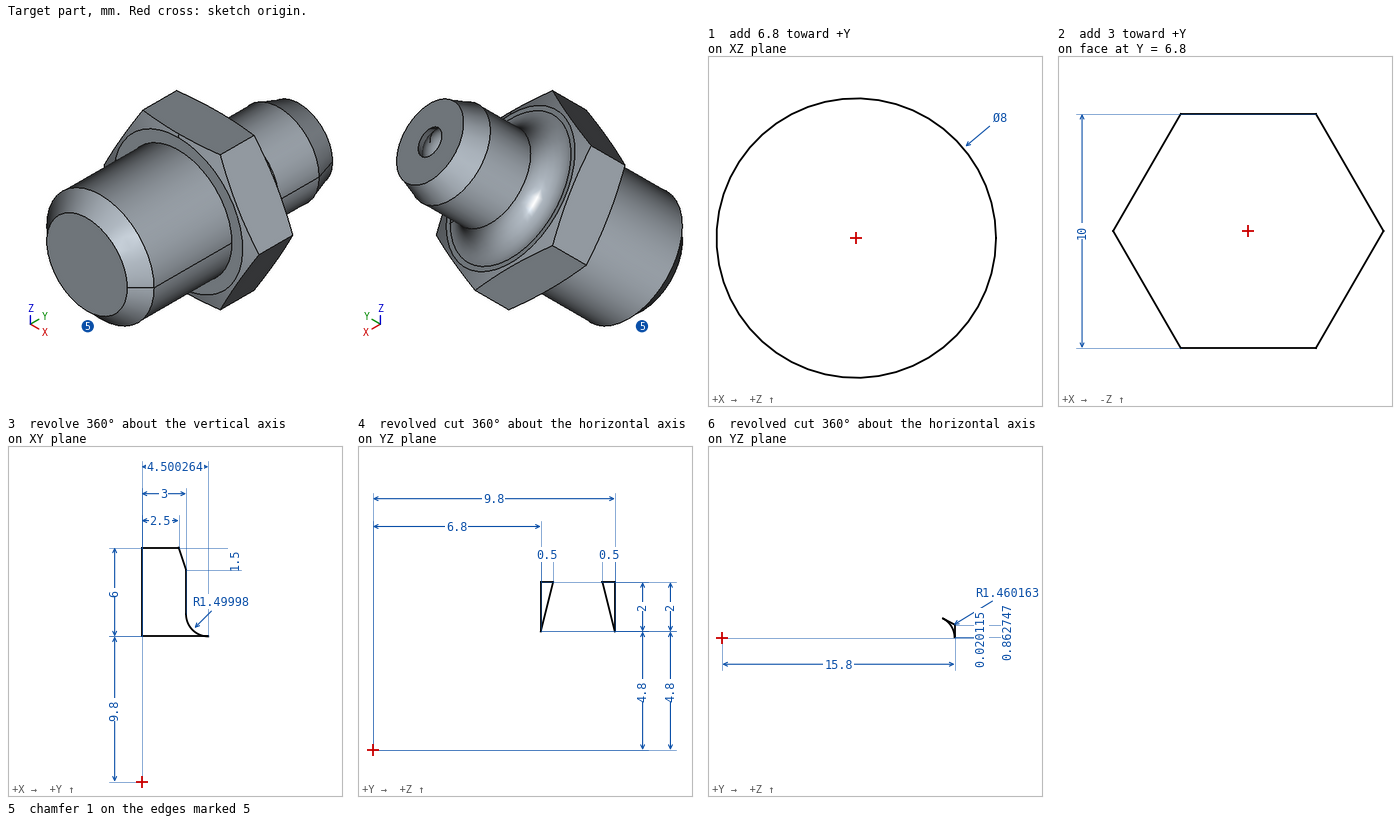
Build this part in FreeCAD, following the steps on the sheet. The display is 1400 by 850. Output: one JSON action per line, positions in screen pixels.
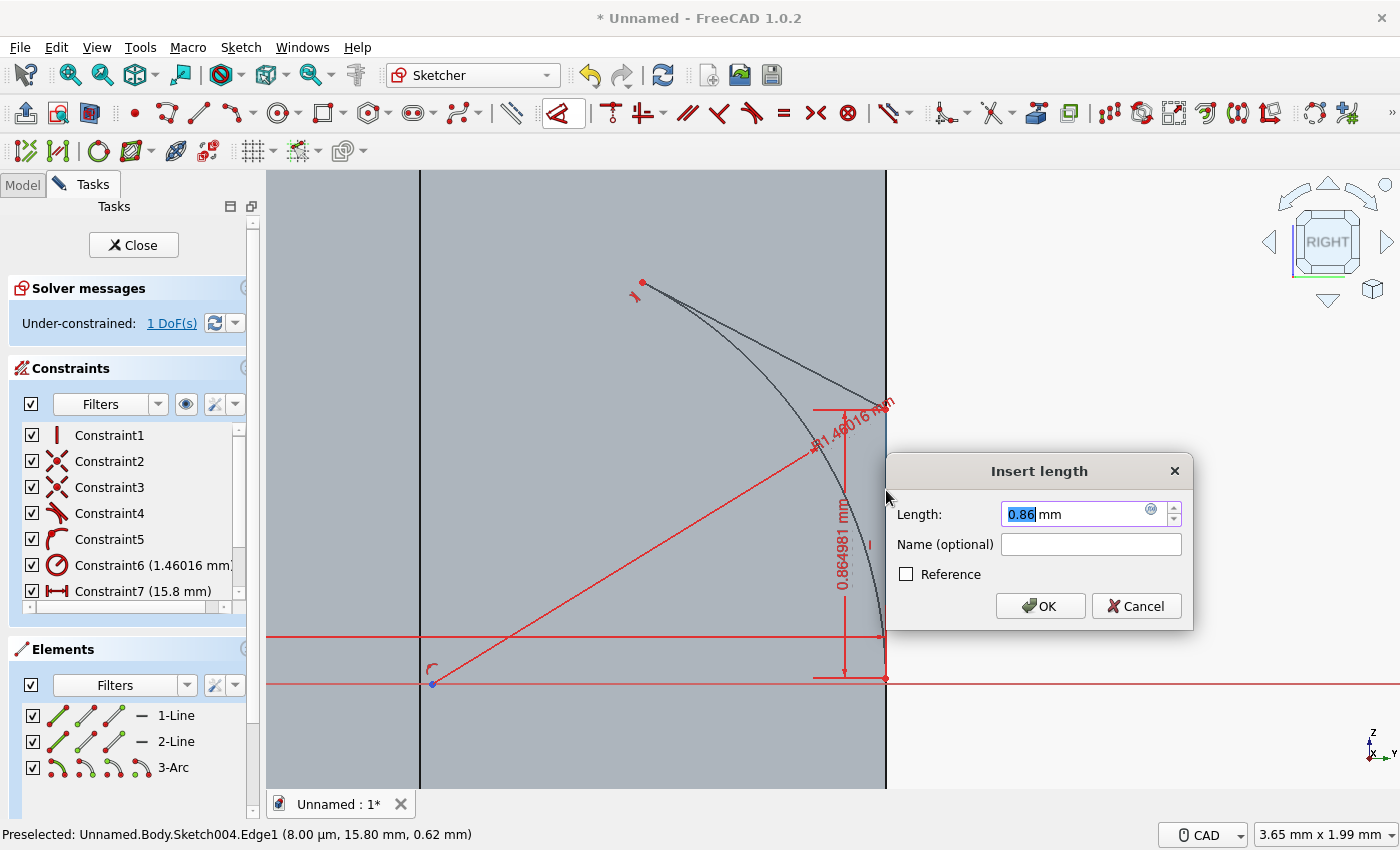
{"action": "type", "text": "0.862747"}
{"action": "key", "text": "Return"}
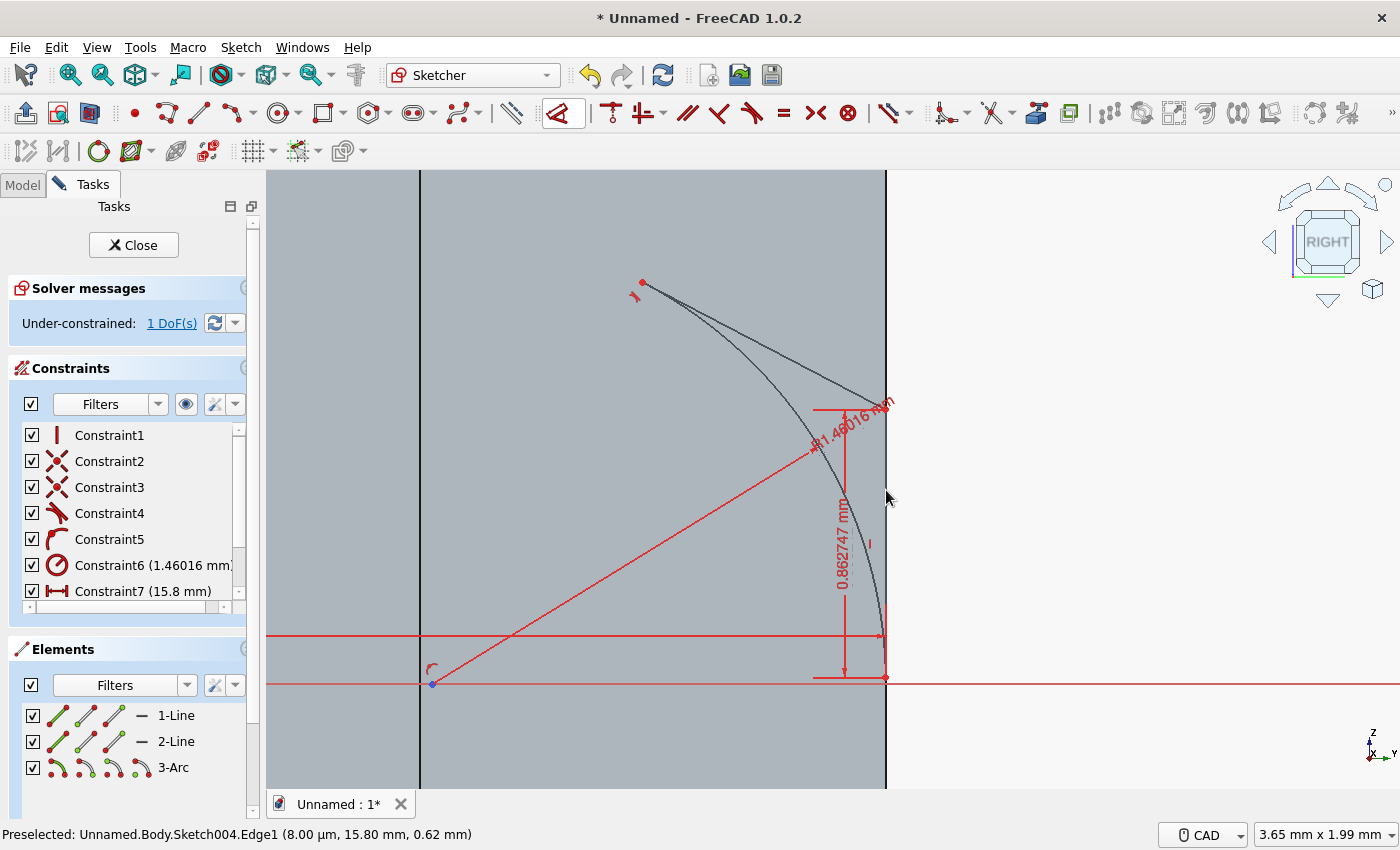
{"action": "scroll", "coordinate": [886, 678], "scroll_direction": "up", "scroll_amount": 10}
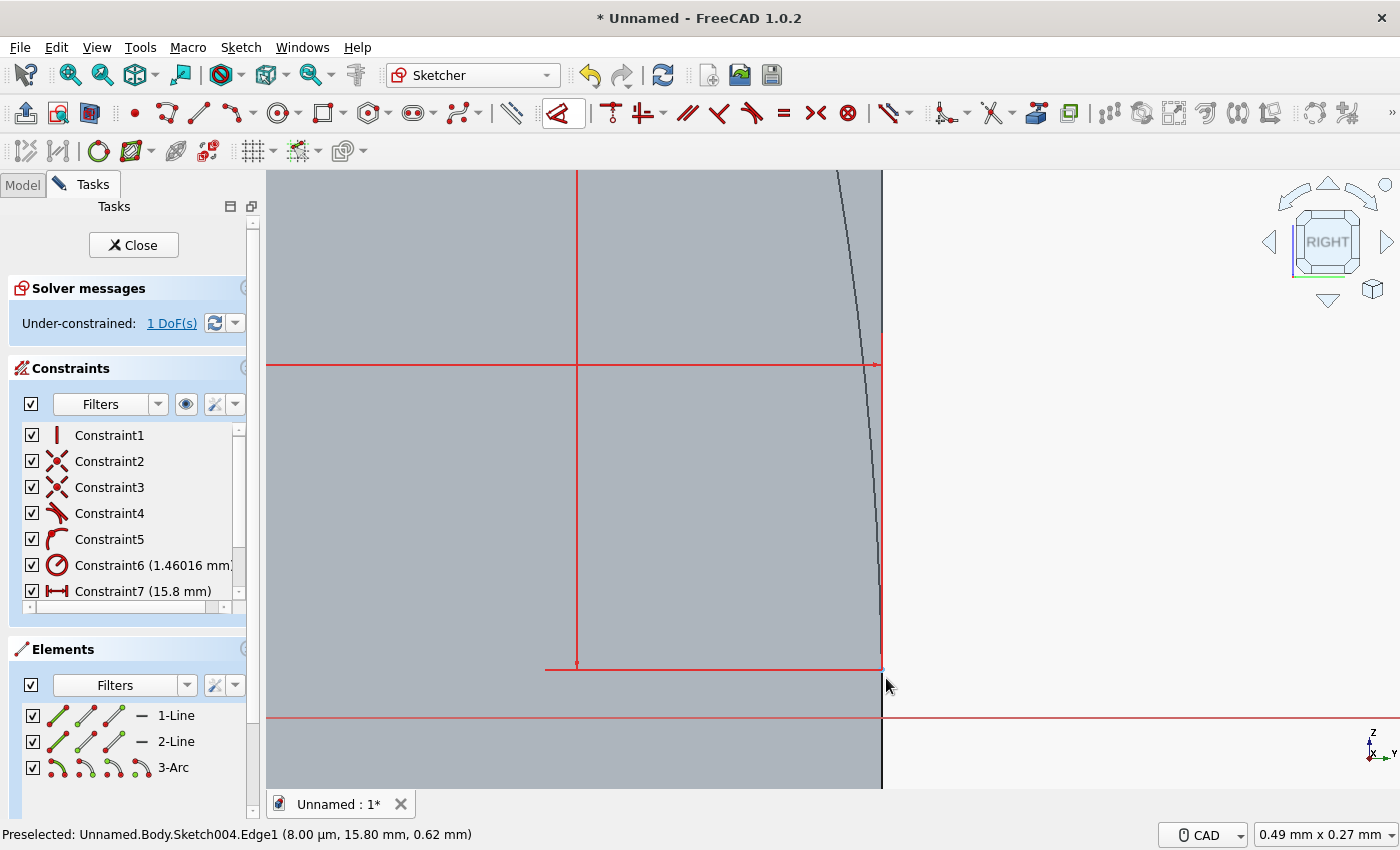
{"action": "left_click", "coordinate": [882, 670]}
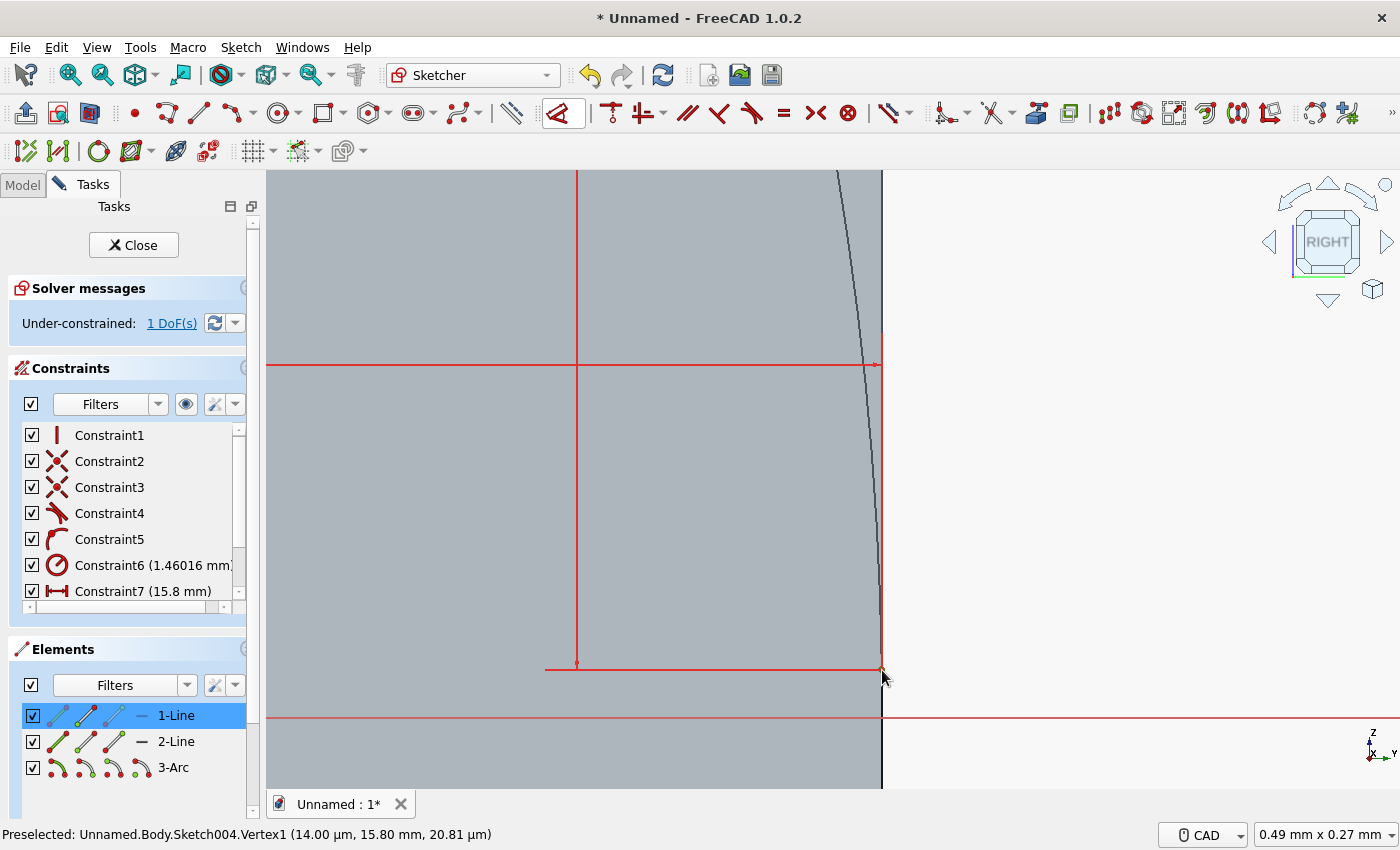
{"action": "key", "text": "i"}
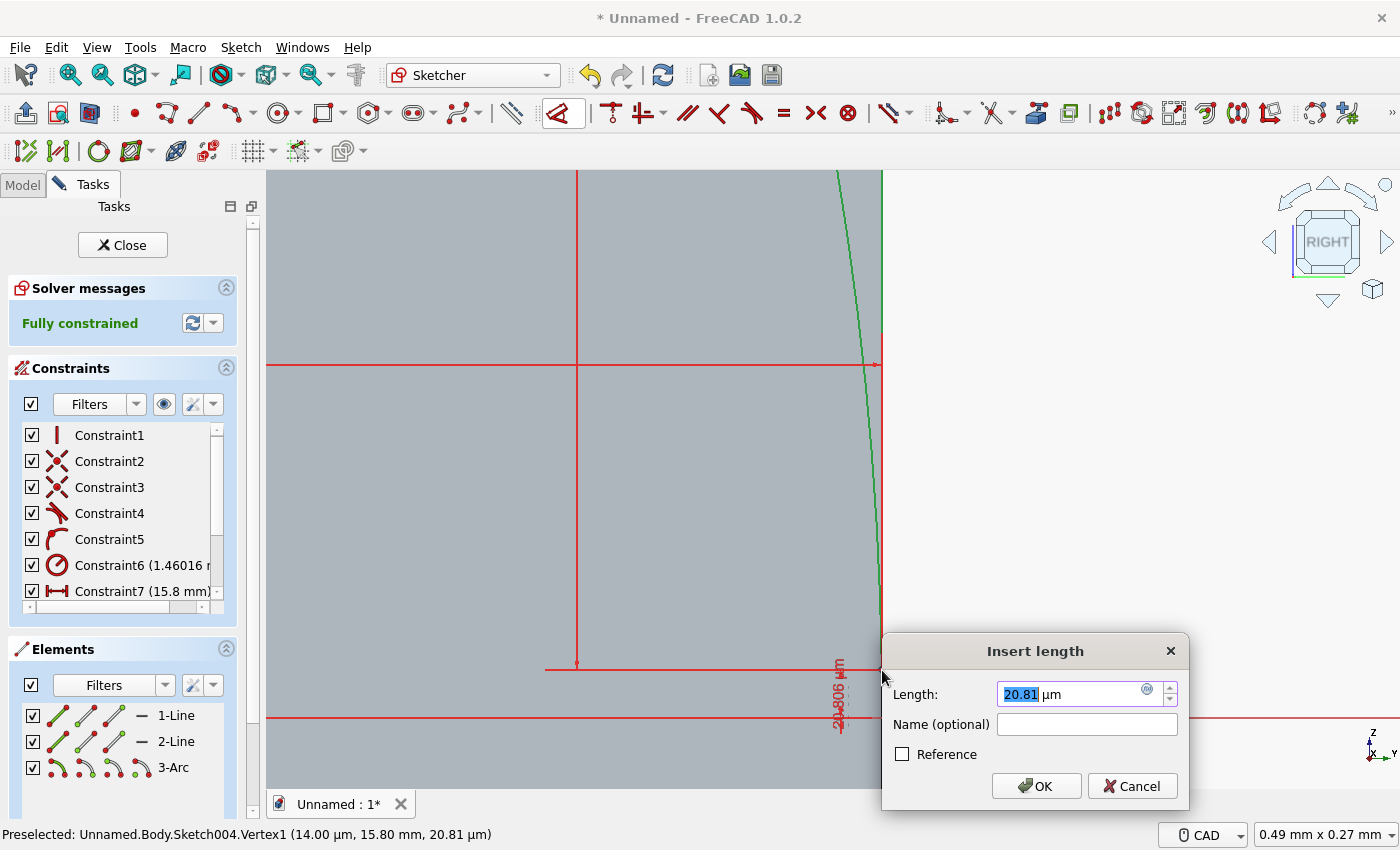
{"action": "key", "text": "ctrl+a"}
{"action": "type", "text": "0.020115 mm"}
{"action": "key", "text": "Return"}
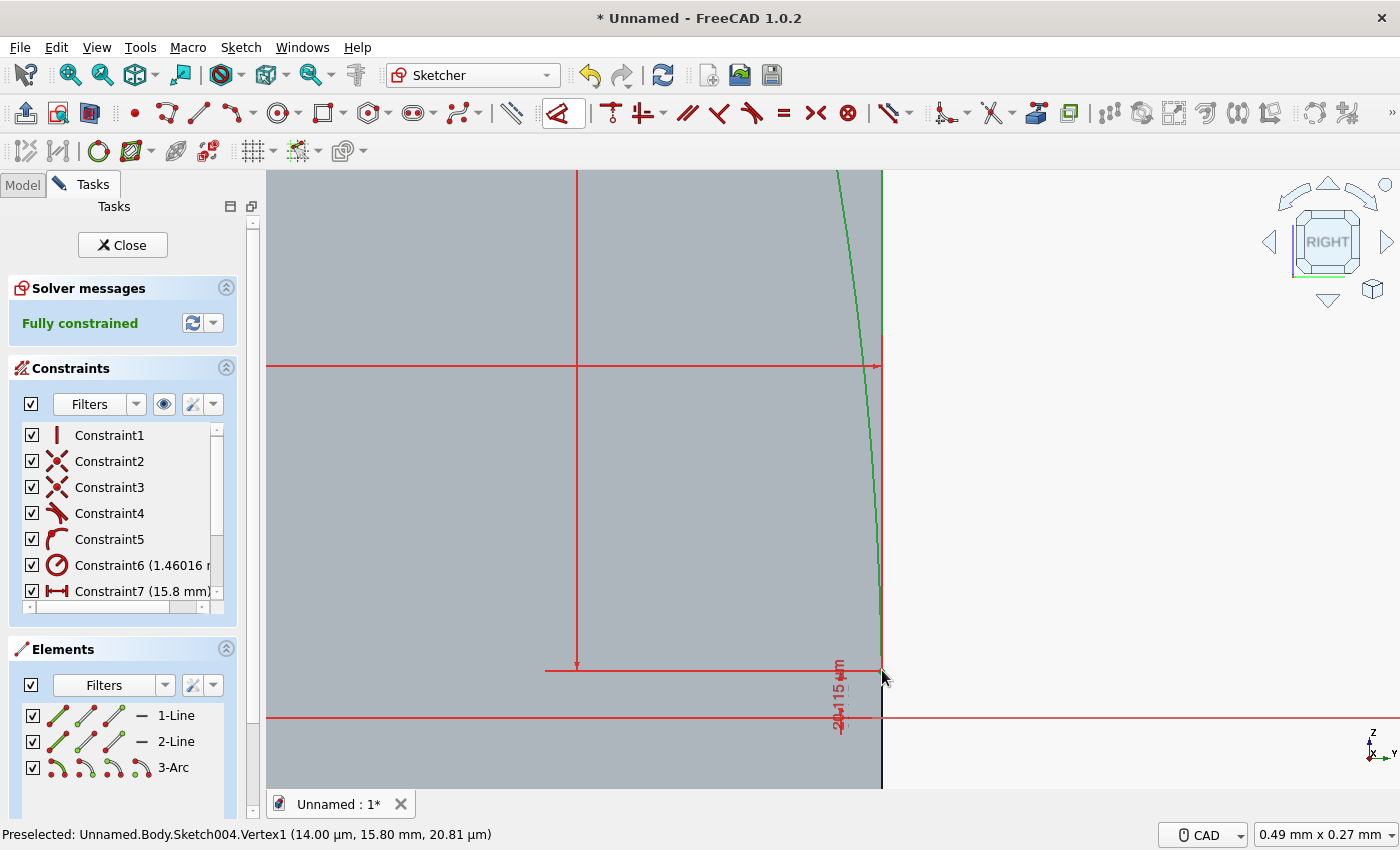
{"action": "left_click", "coordinate": [123, 245]}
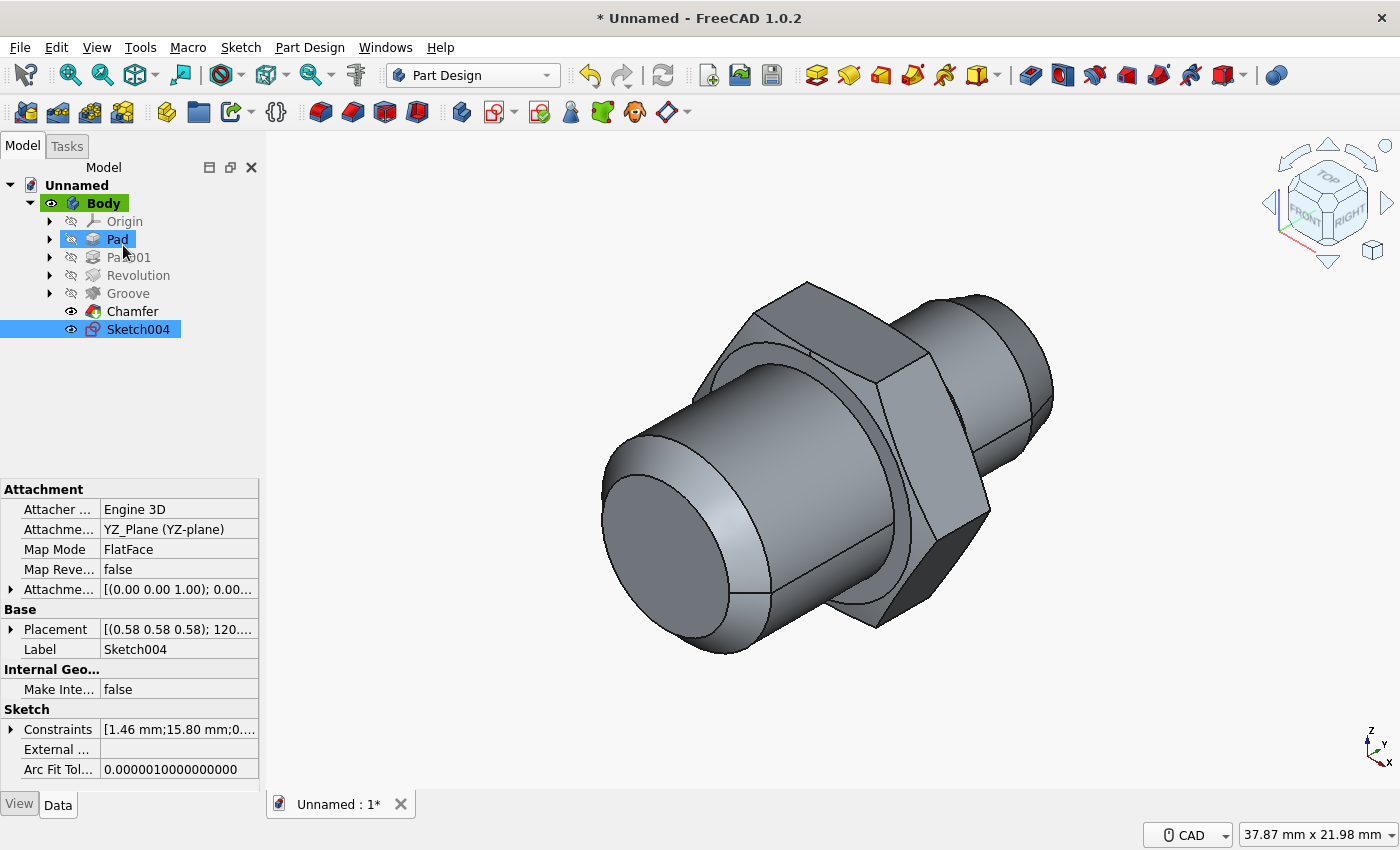
{"action": "left_click", "coordinate": [1096, 76]}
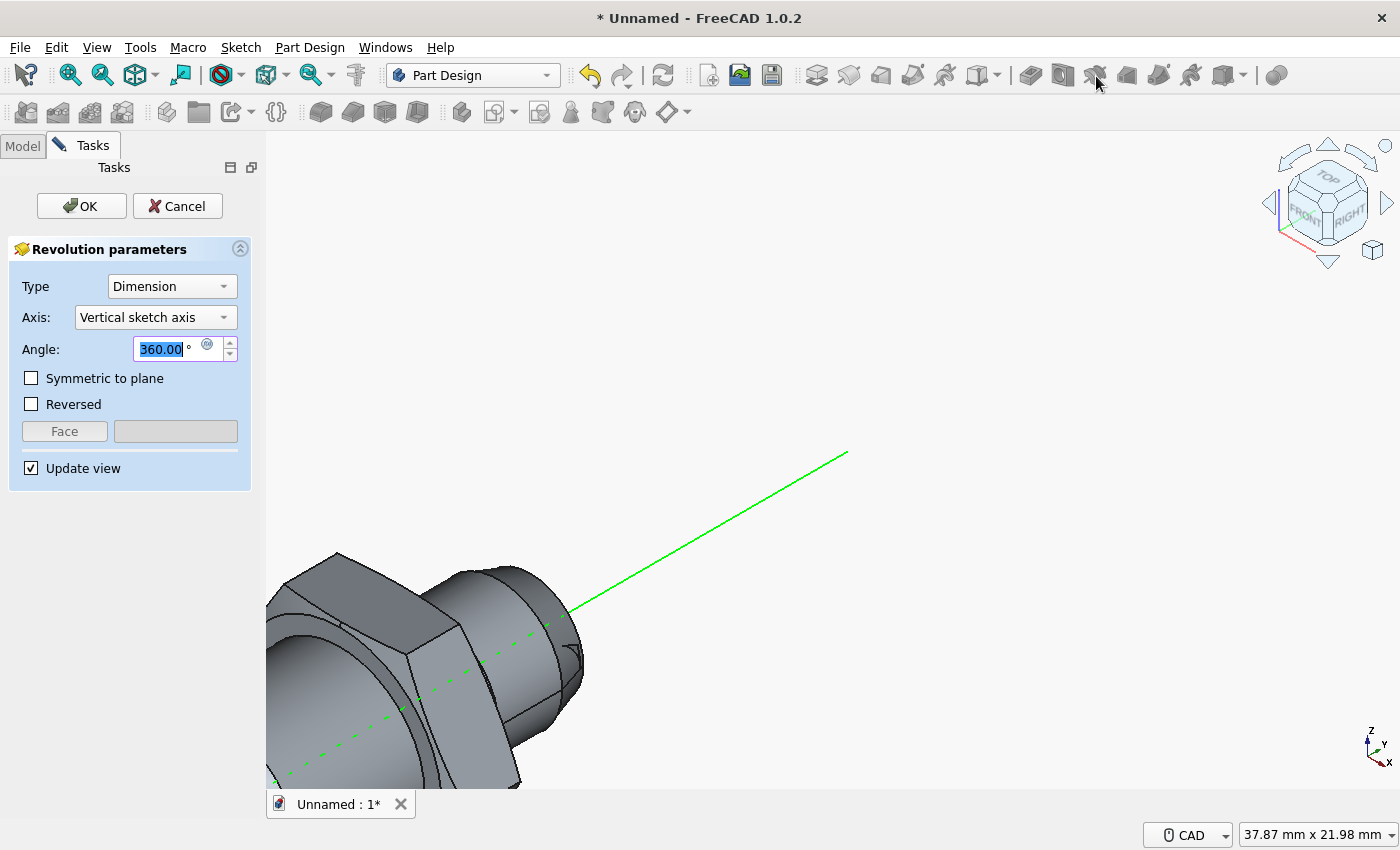
{"action": "left_click", "coordinate": [156, 318]}